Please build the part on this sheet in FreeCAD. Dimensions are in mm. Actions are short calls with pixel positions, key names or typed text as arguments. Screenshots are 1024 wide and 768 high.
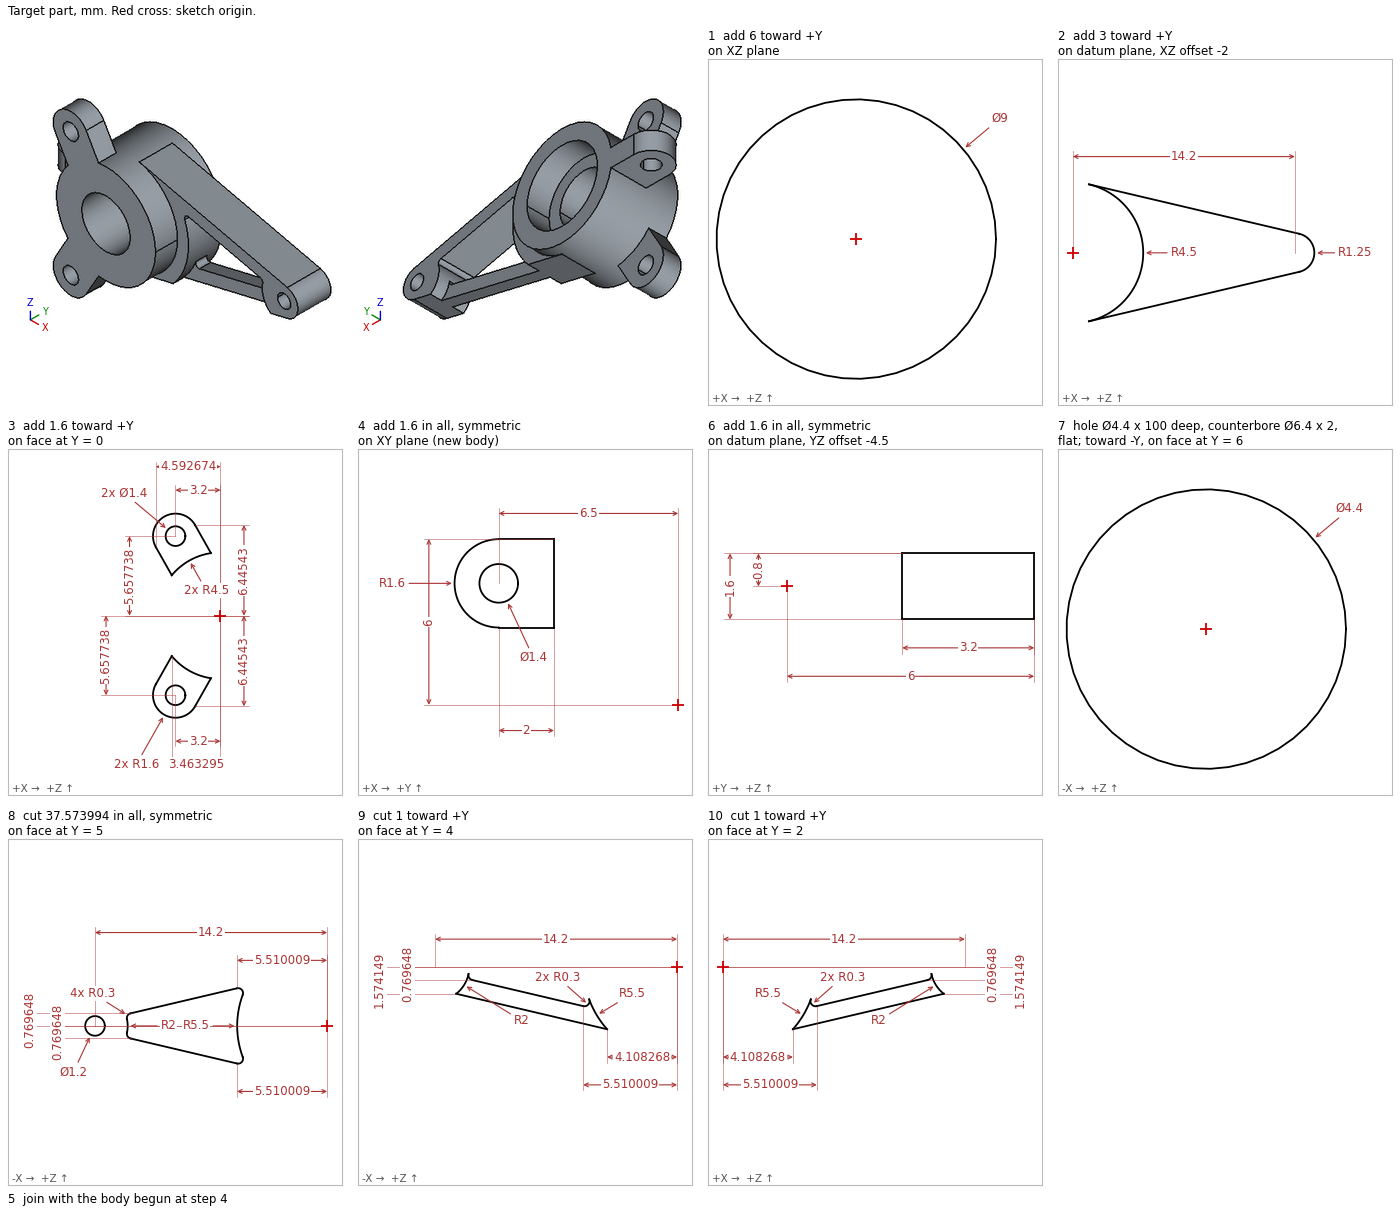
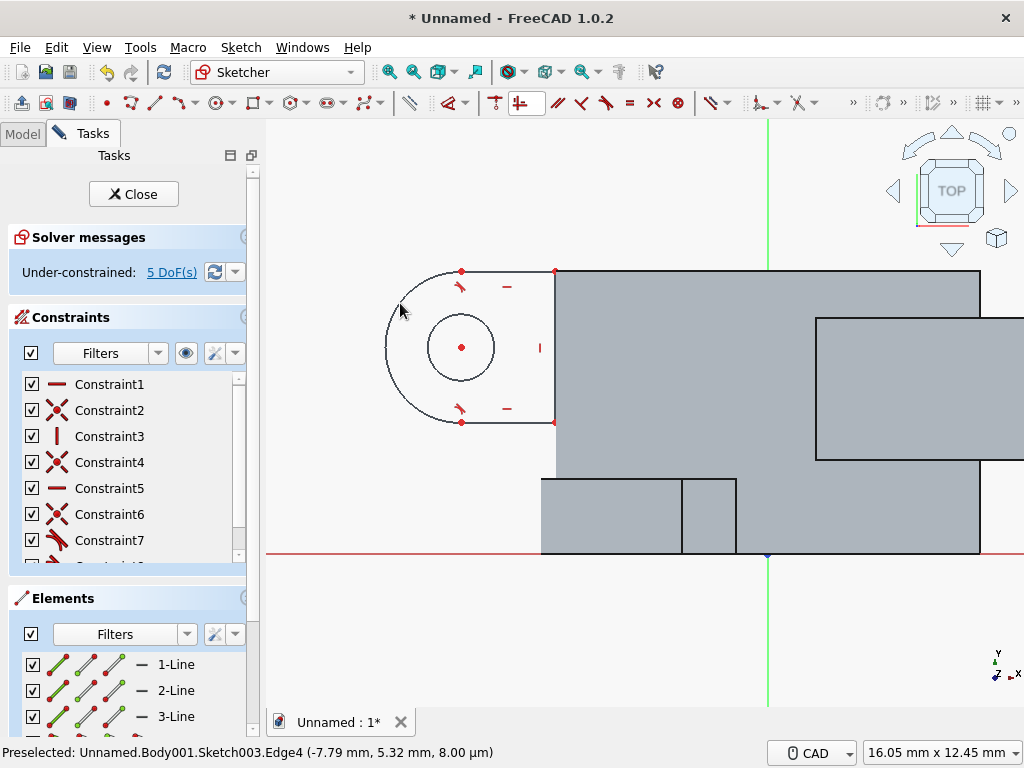
click(448, 104)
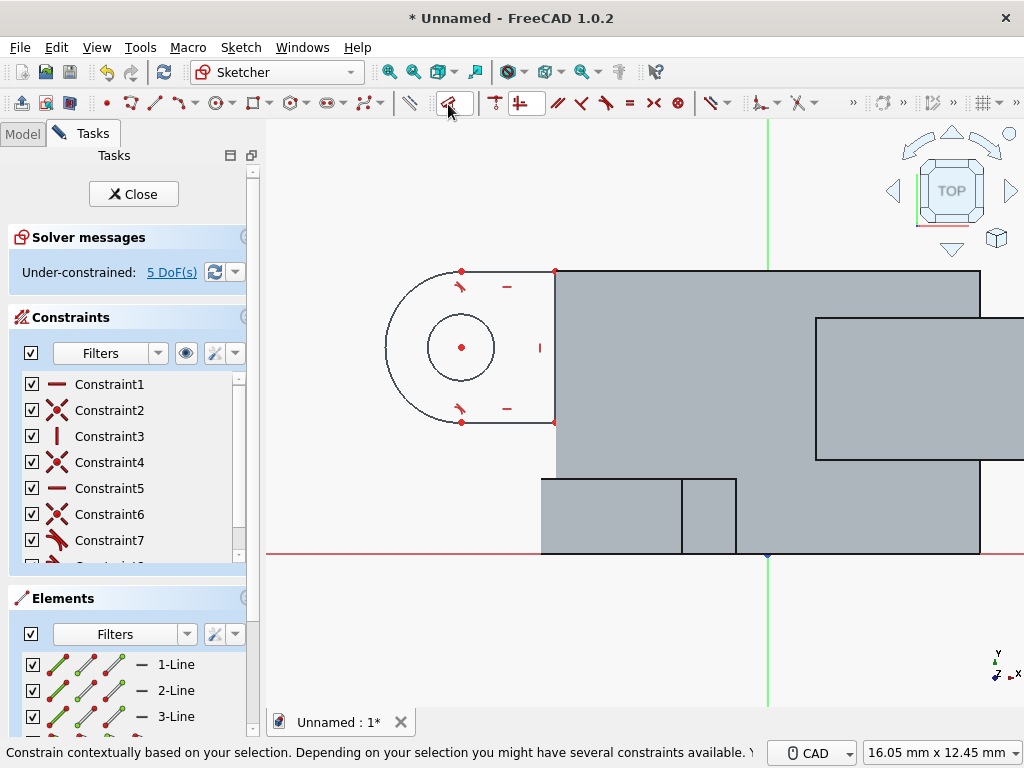
click(400, 303)
click(374, 284)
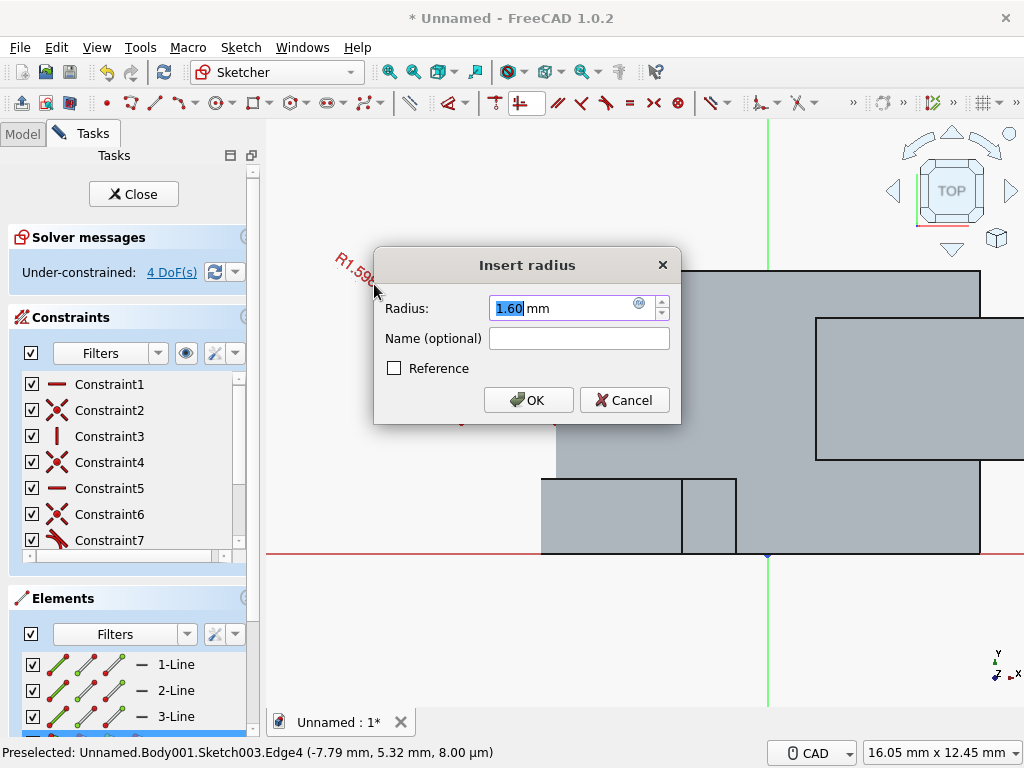
text(1.6)
key(Return)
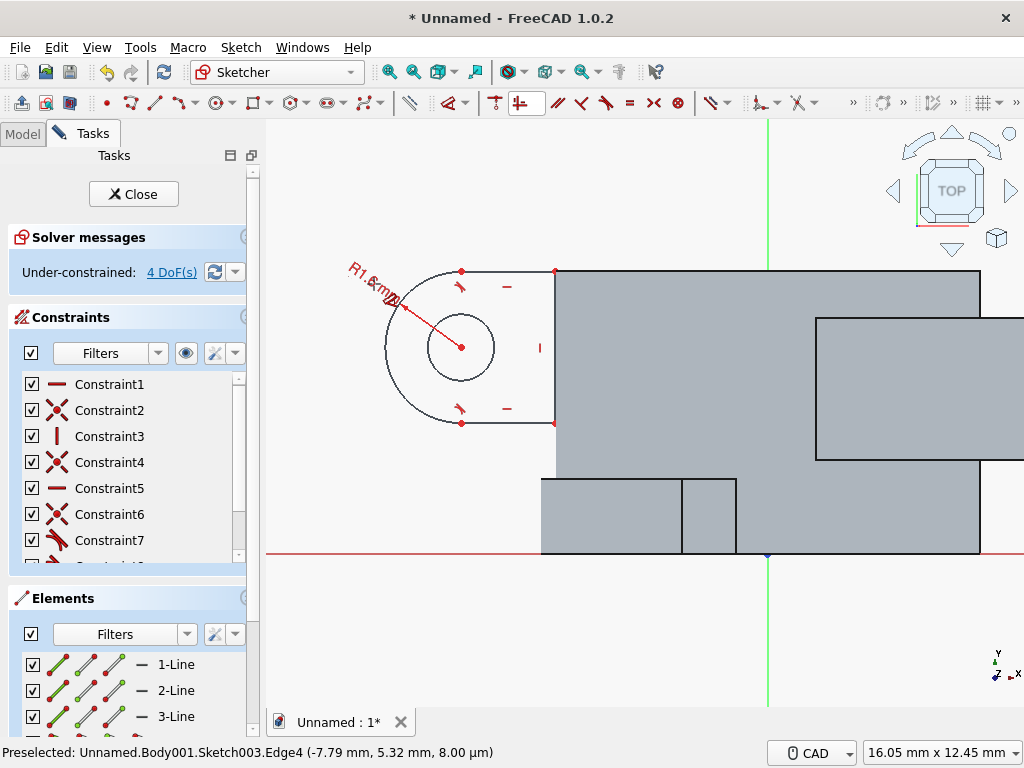
click(484, 324)
click(506, 301)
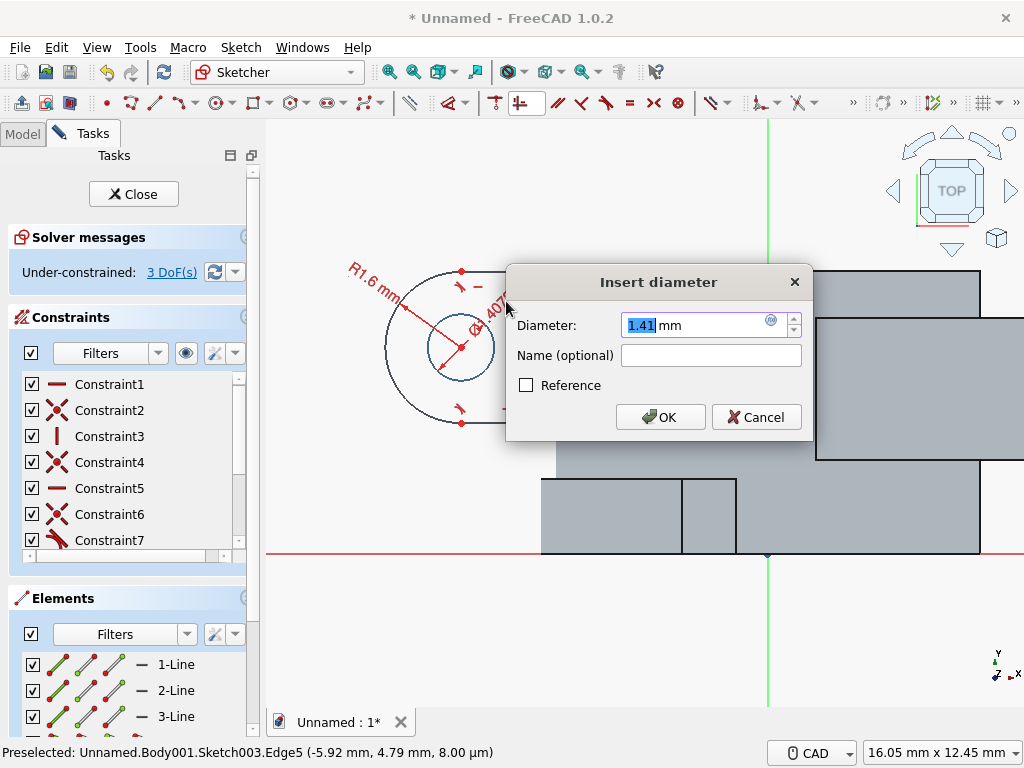
text(1.4)
key(Return)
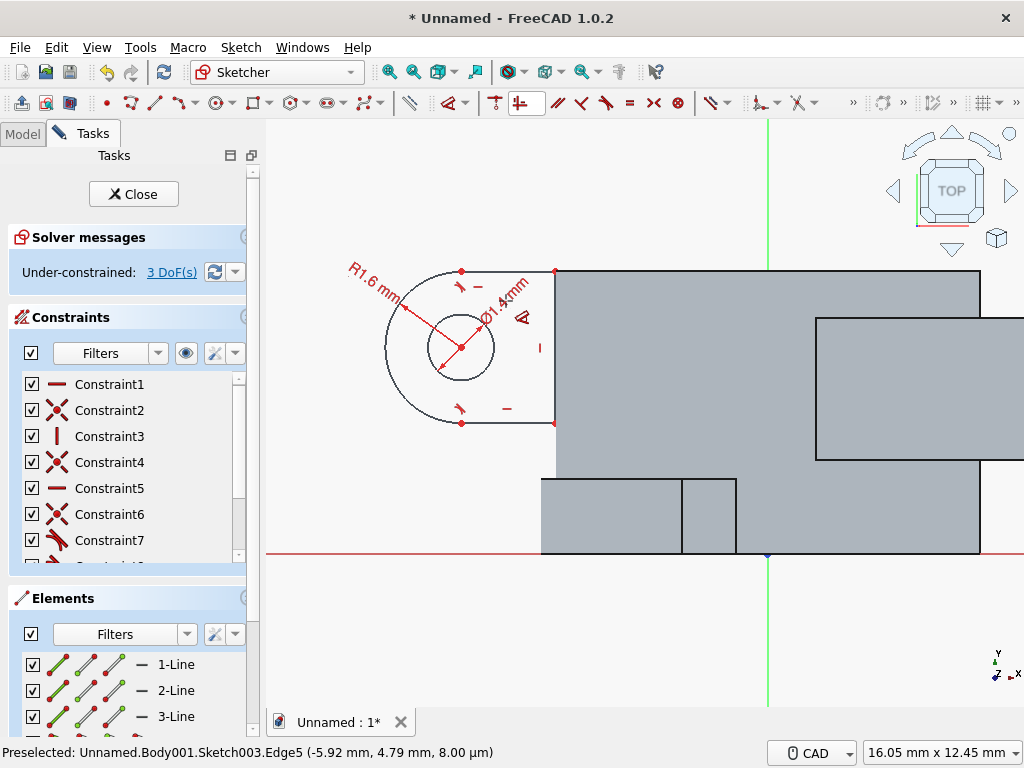
click(489, 423)
click(508, 457)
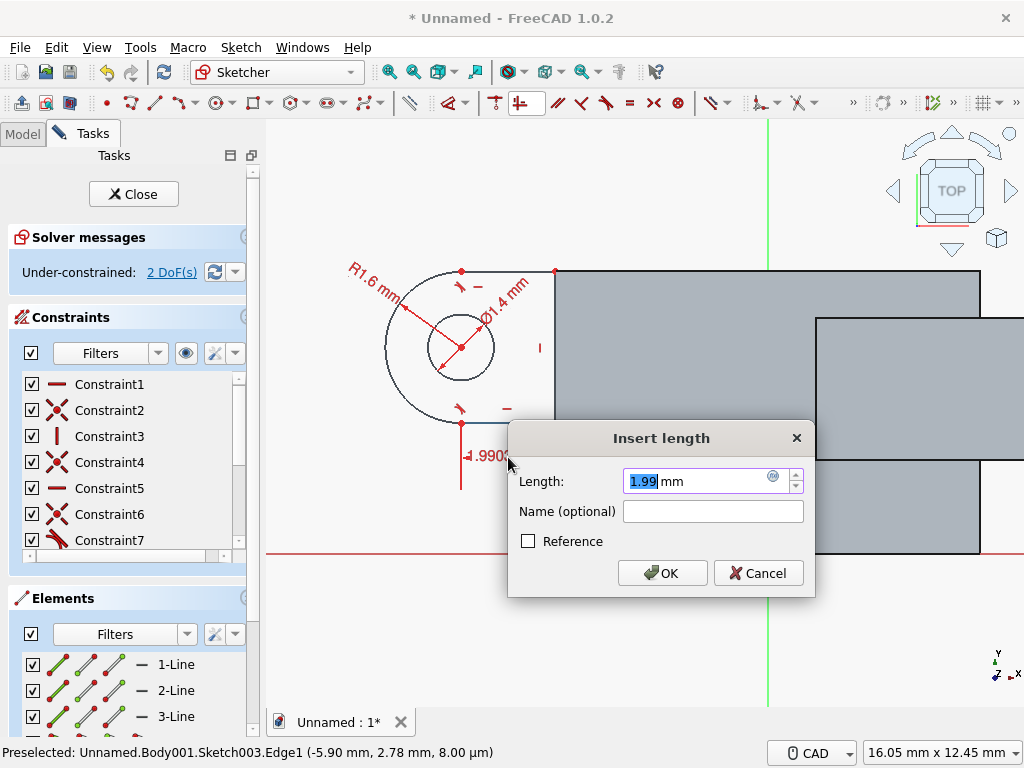
text(2)
key(Return)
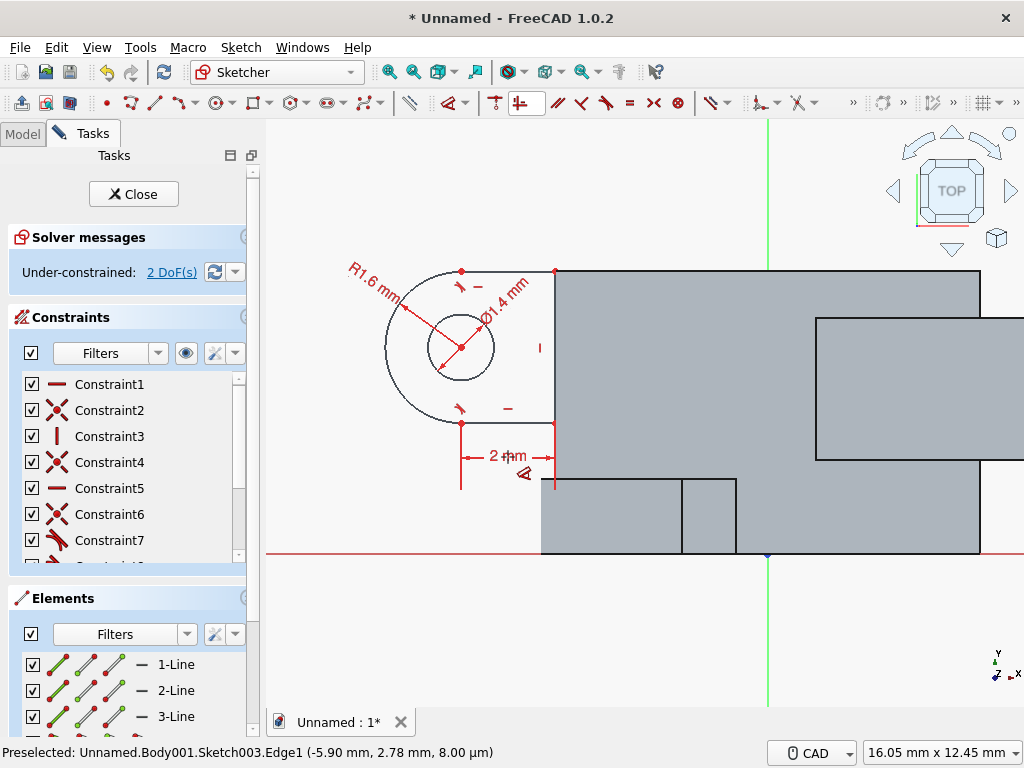
click(555, 272)
click(802, 413)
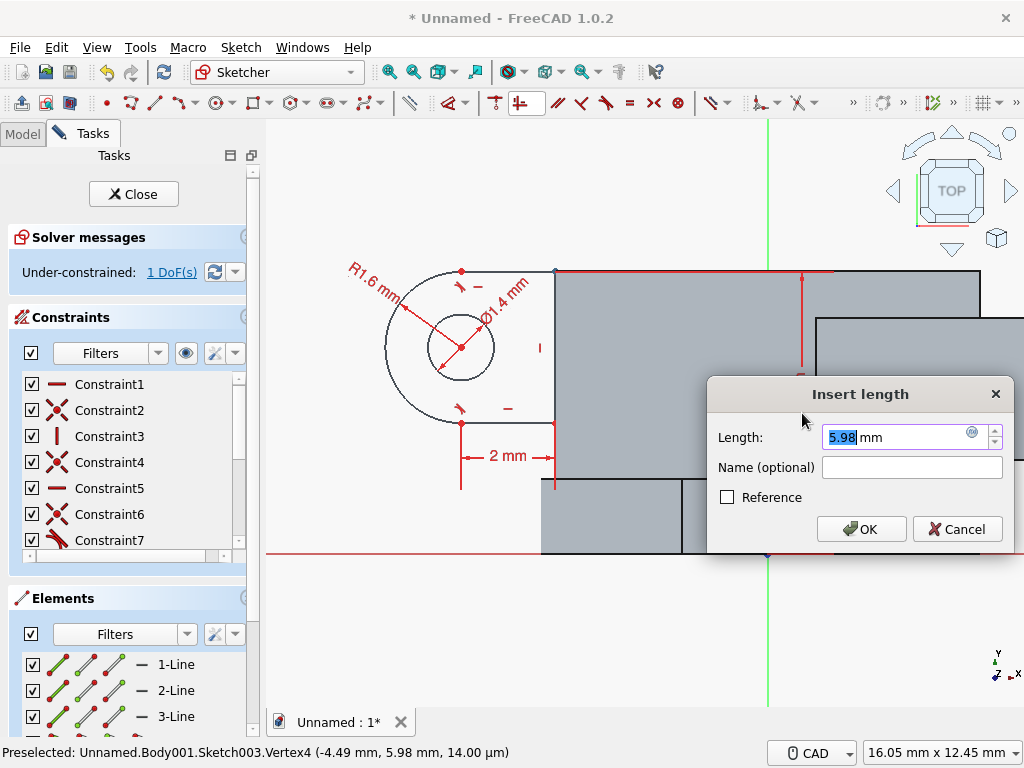
text(6)
key(Return)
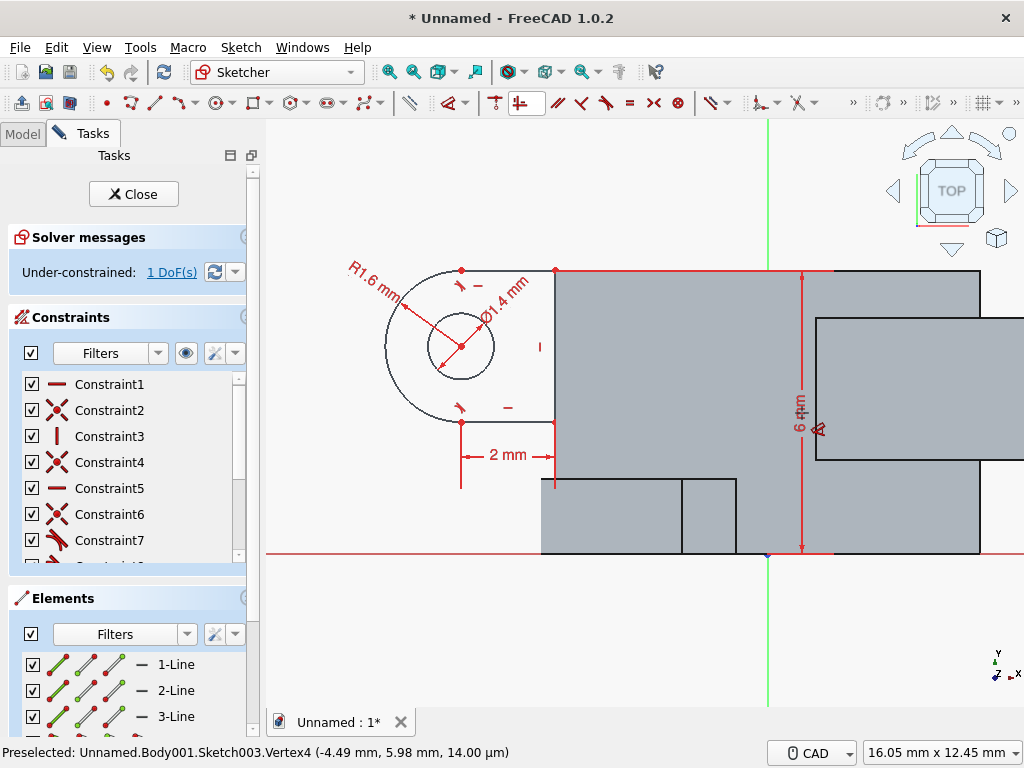
click(461, 346)
click(614, 588)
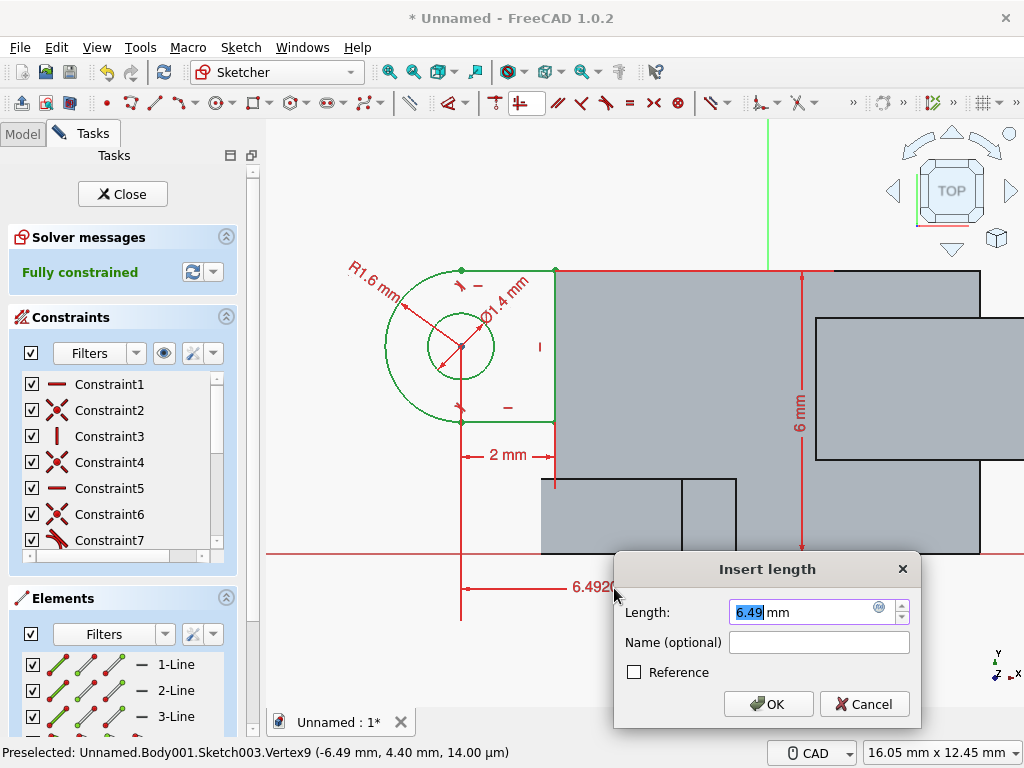
text(6.5)
key(Return)
key(Escape)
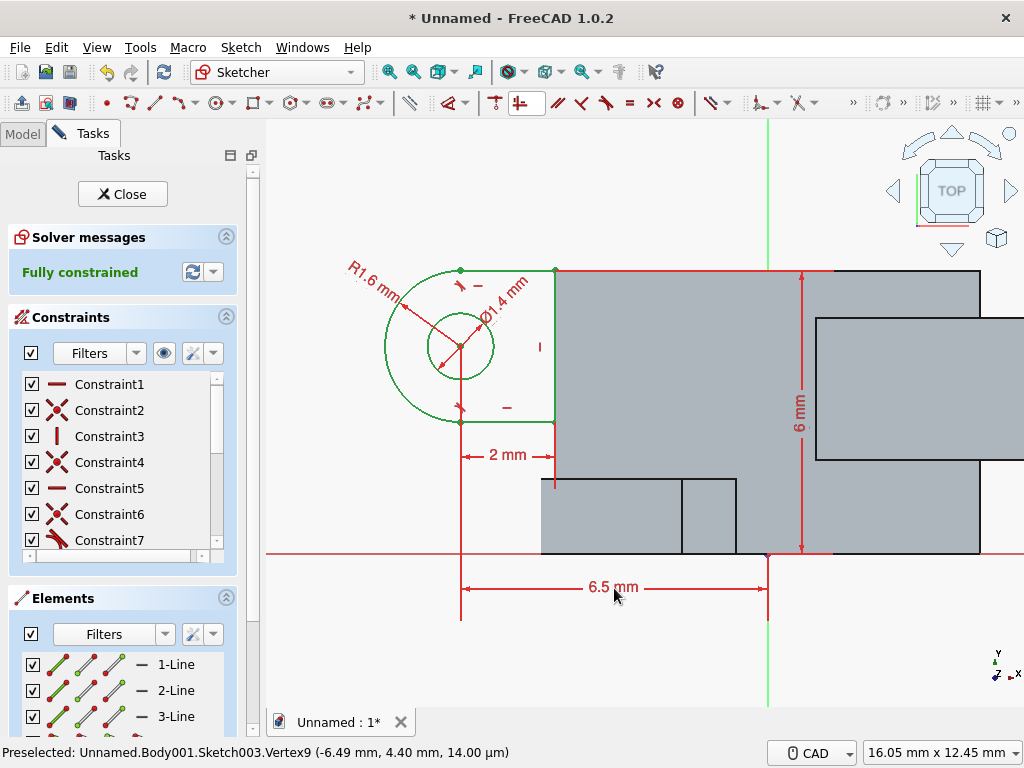
click(123, 194)